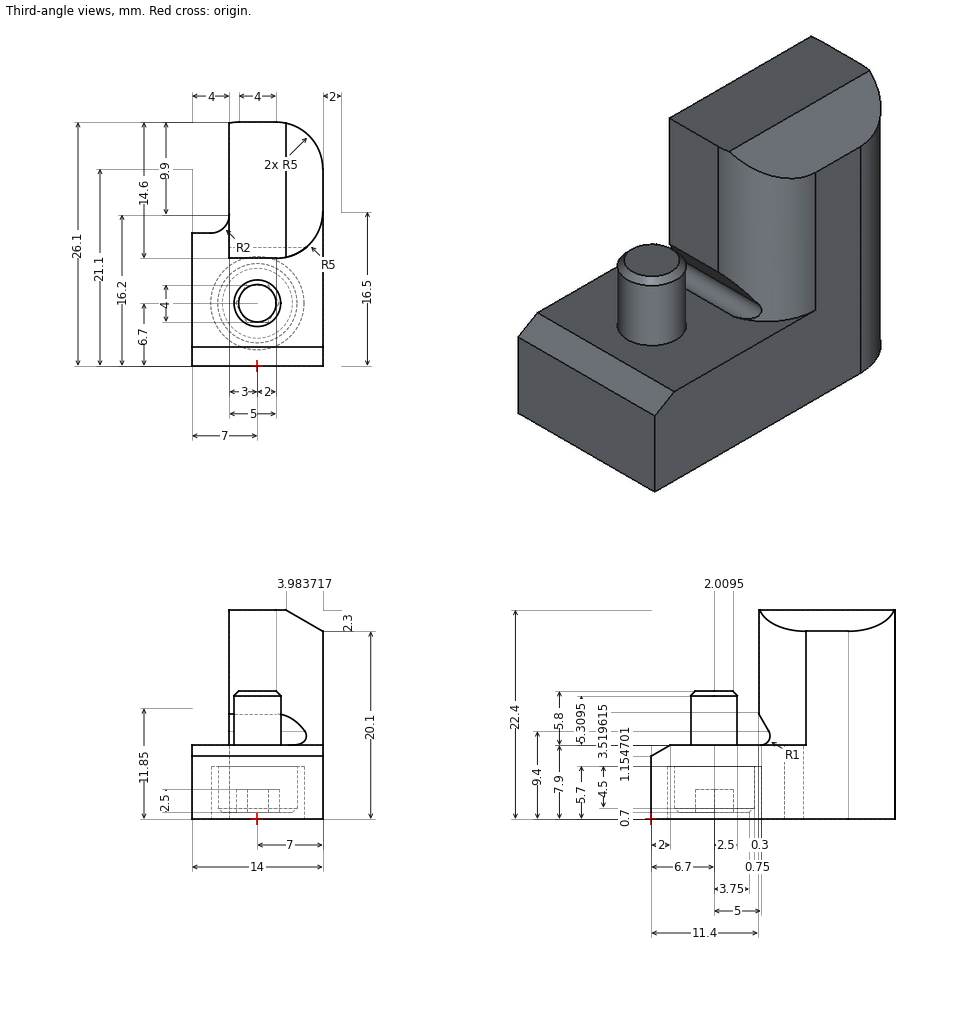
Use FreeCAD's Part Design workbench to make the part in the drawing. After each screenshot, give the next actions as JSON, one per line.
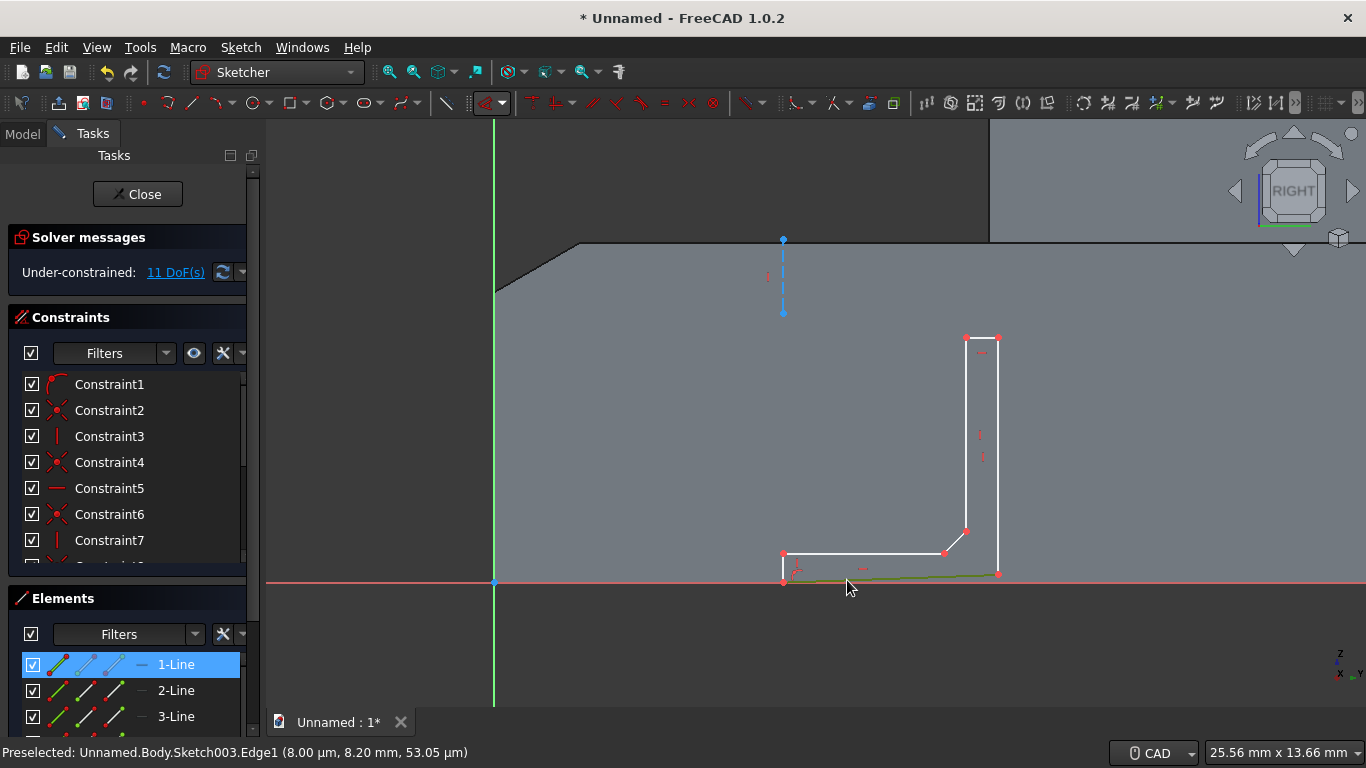
{"action": "key", "text": "h"}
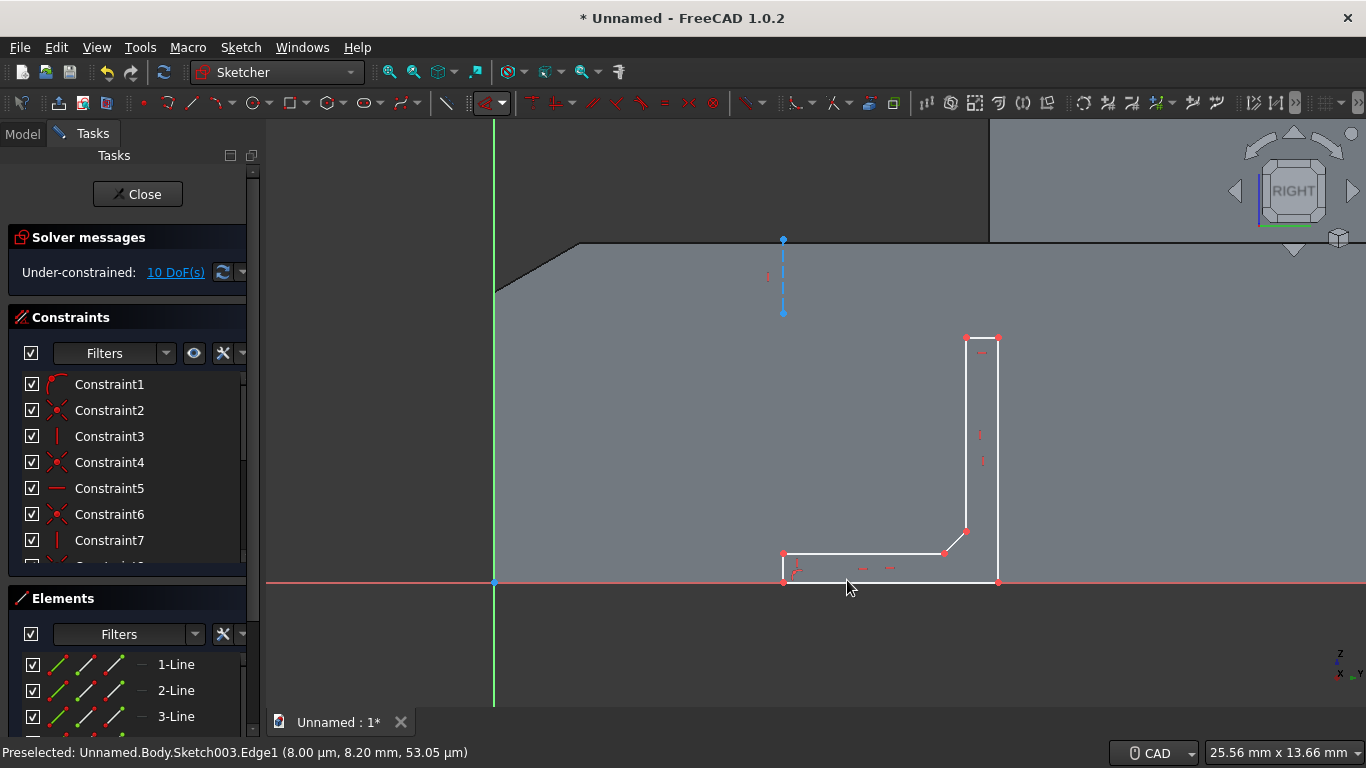
{"action": "left_click", "coordinate": [847, 583]}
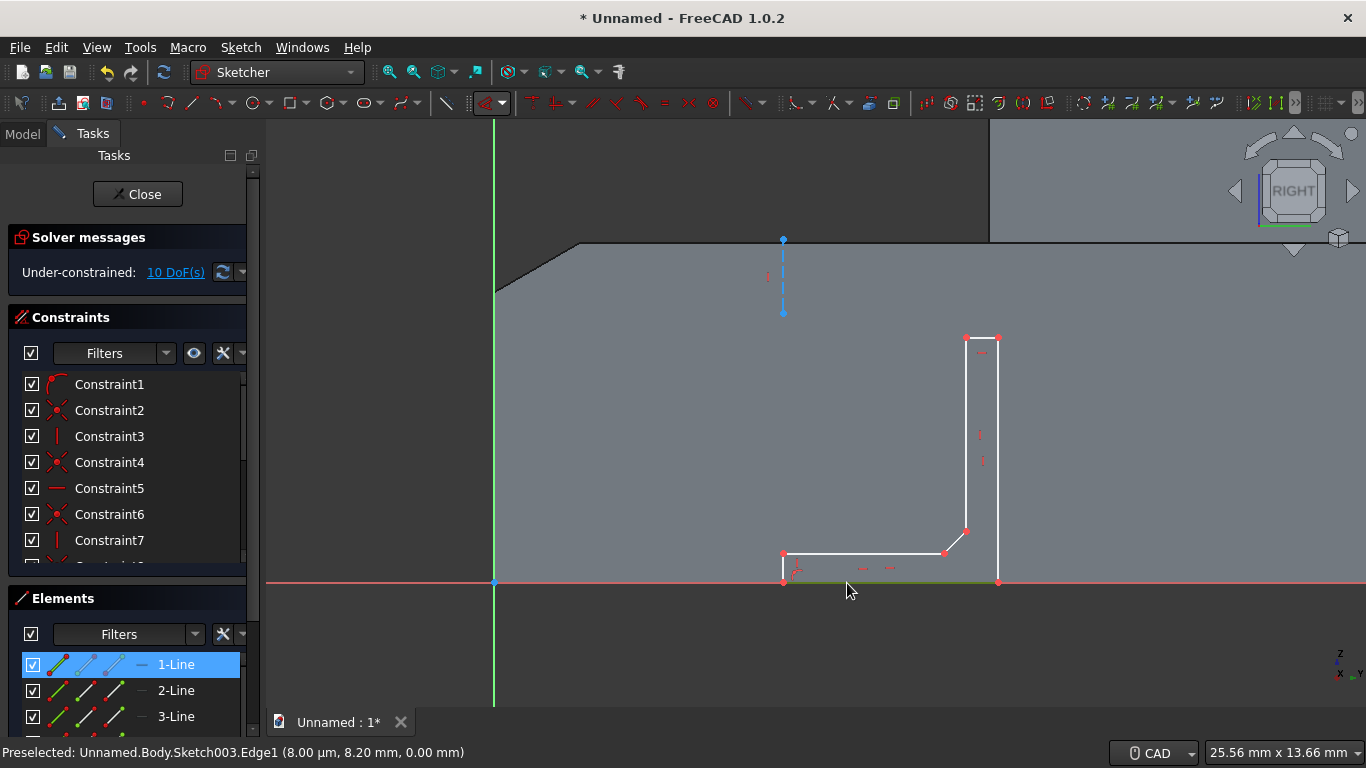
{"action": "key", "text": "l"}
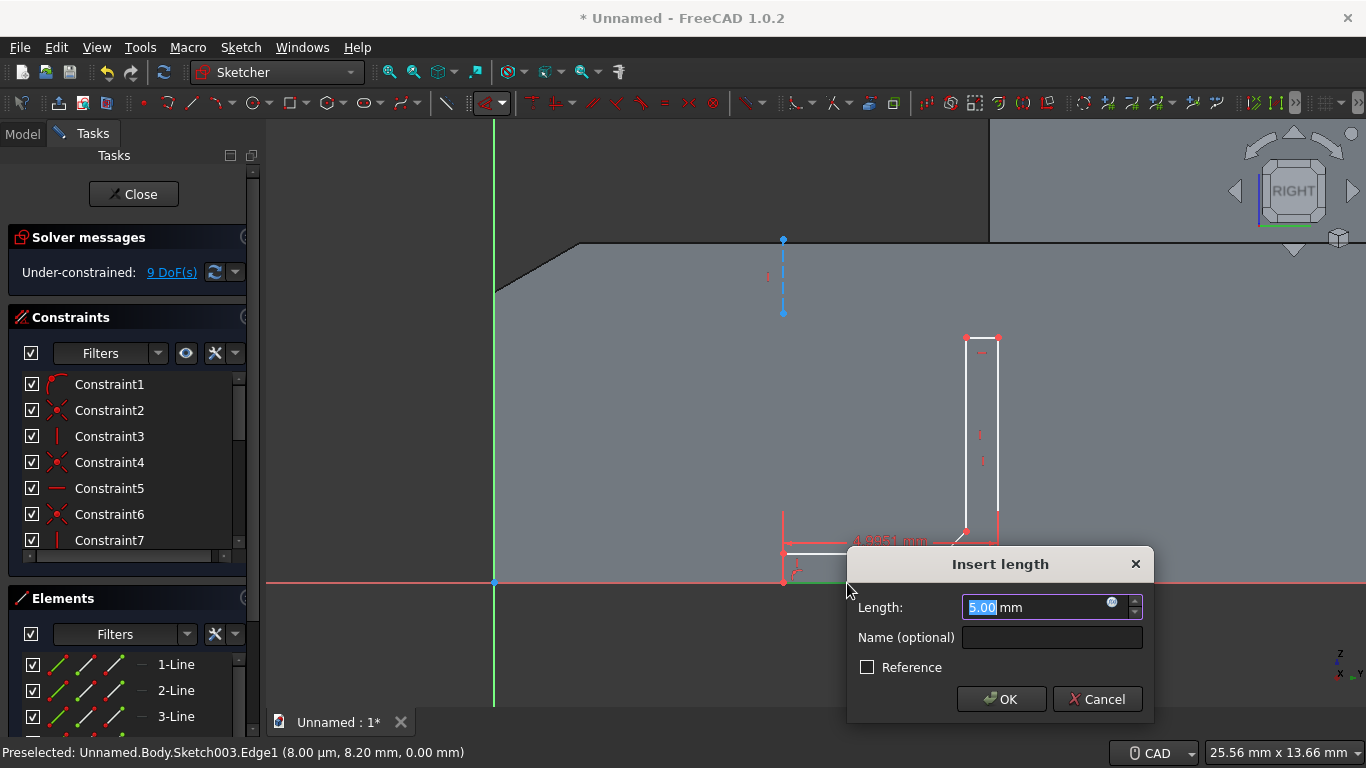
{"action": "type", "text": "5"}
{"action": "key", "text": "Return"}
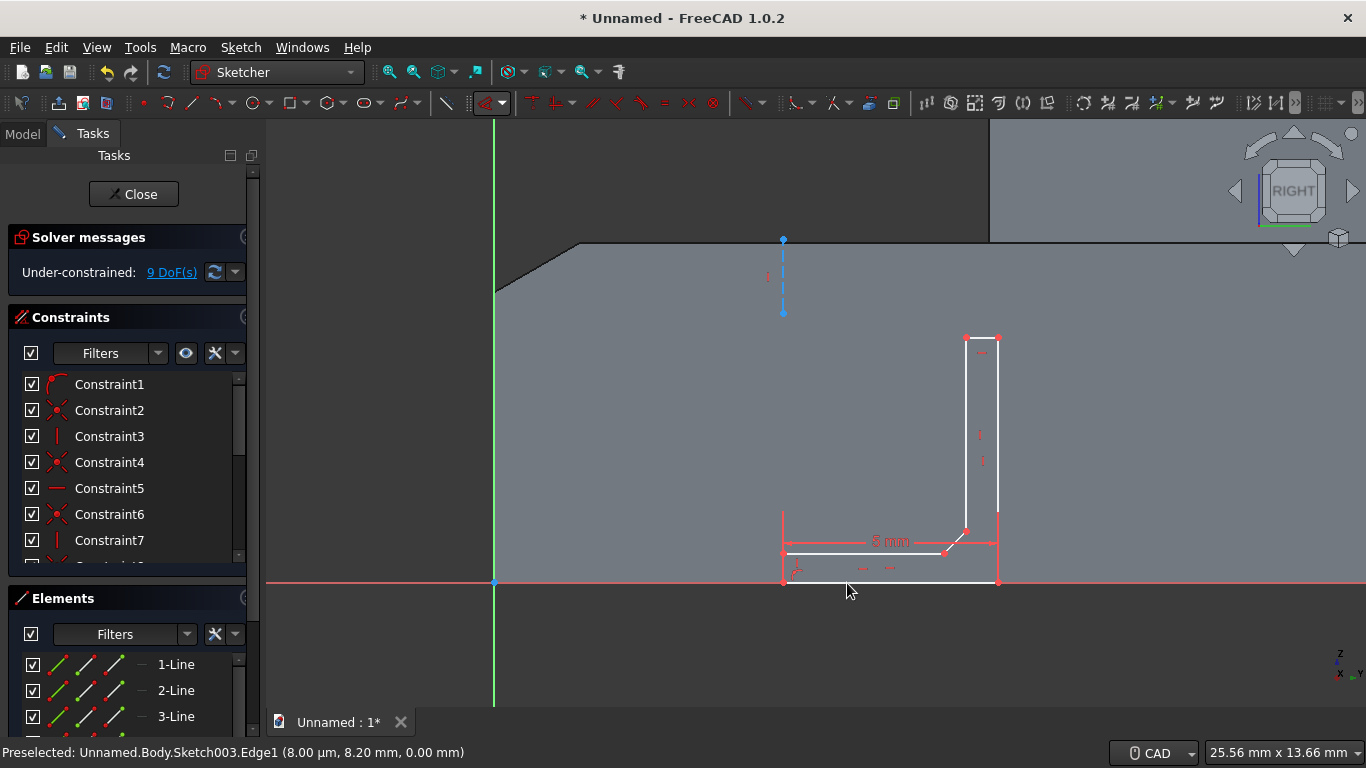
{"action": "left_click", "coordinate": [998, 509]}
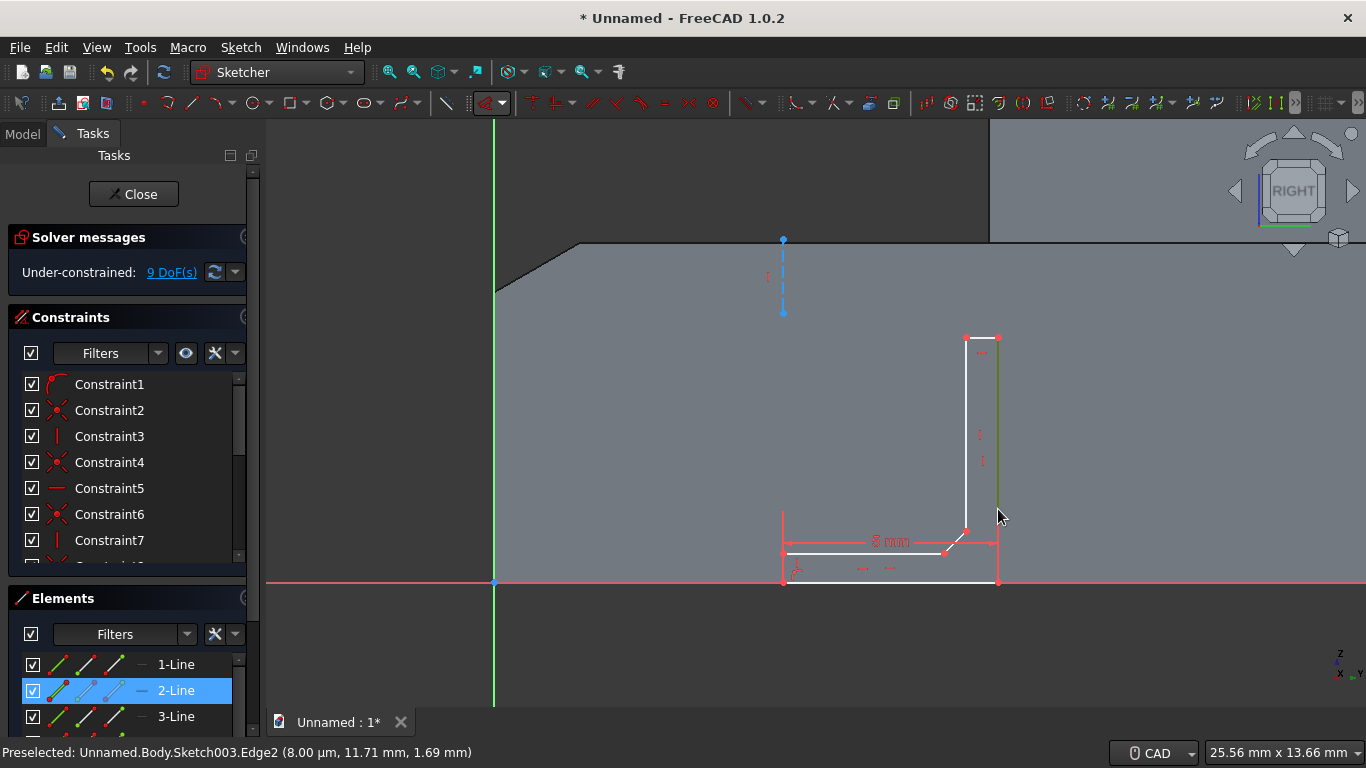
{"action": "left_click", "coordinate": [504, 104]}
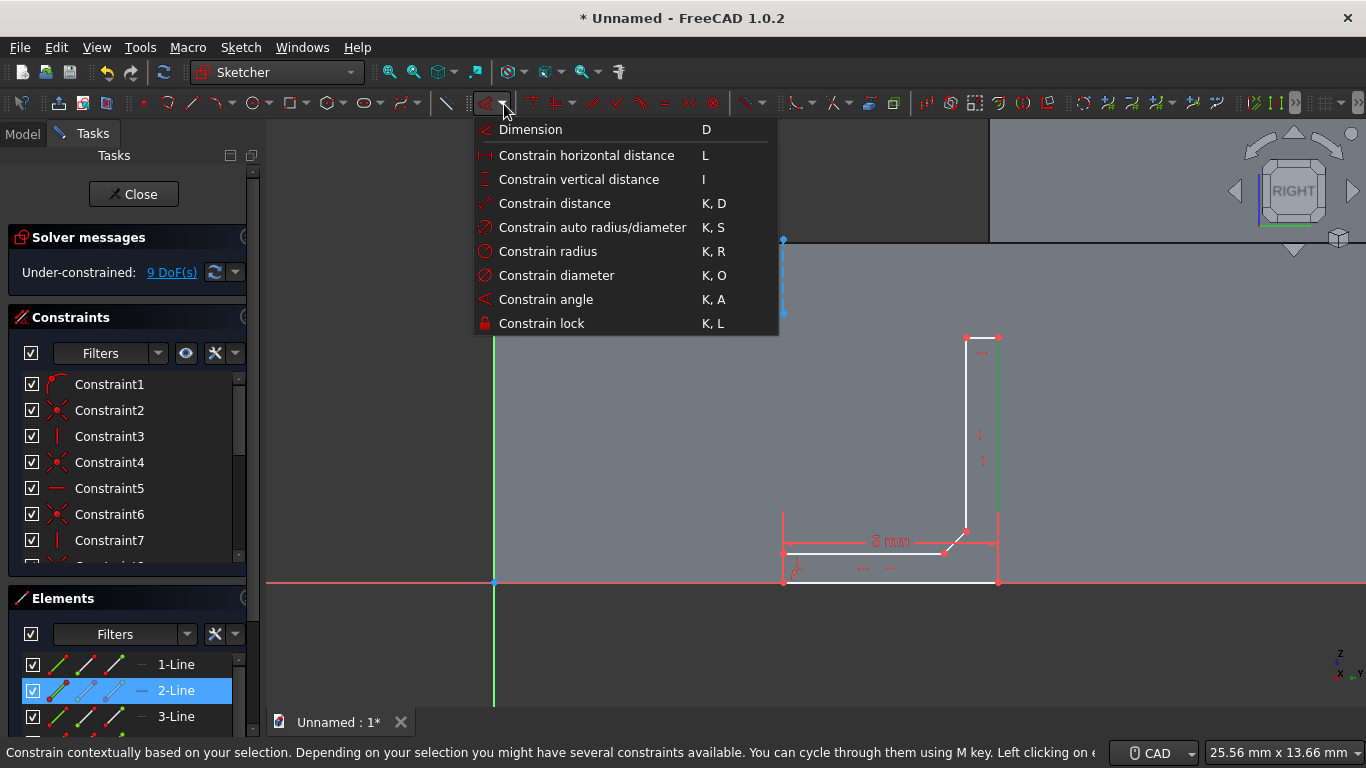
{"action": "left_click", "coordinate": [626, 179]}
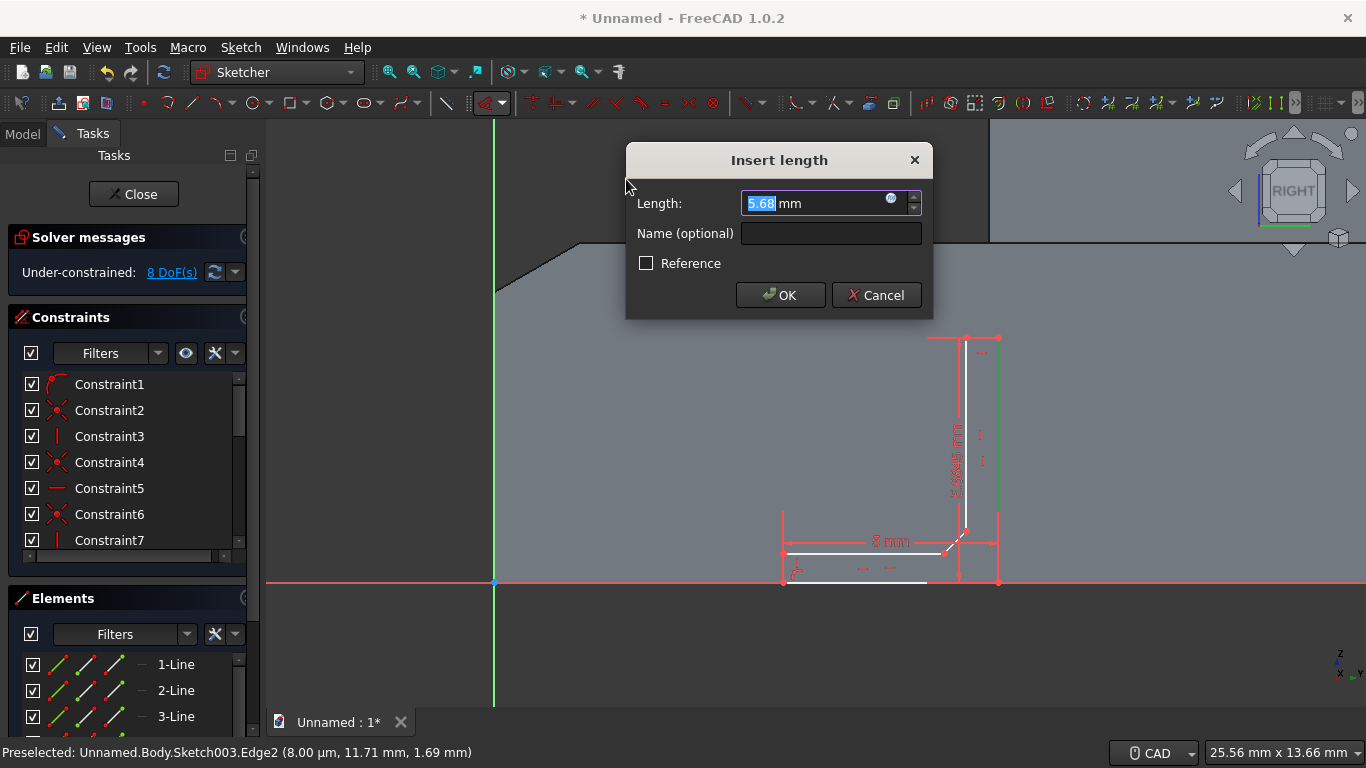
{"action": "type", "text": "5.7"}
{"action": "key", "text": "Return"}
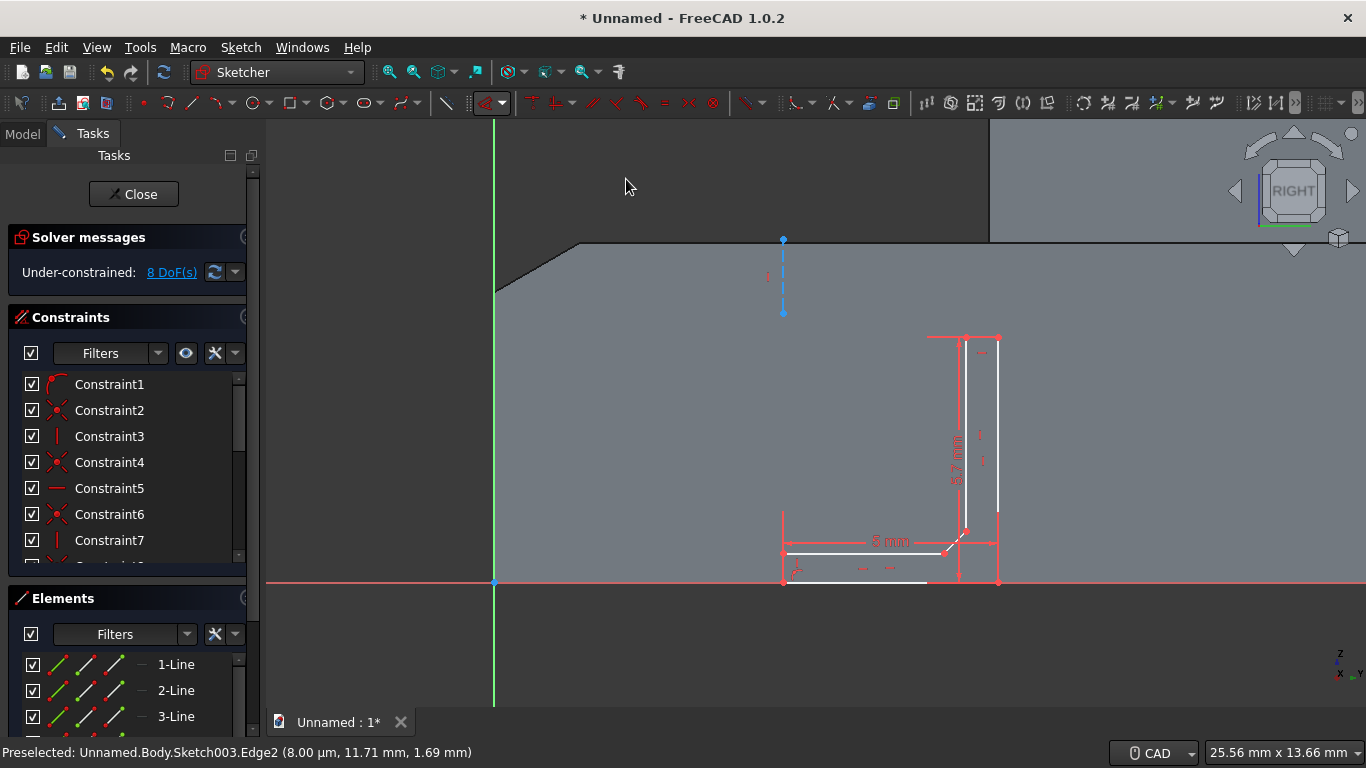
{"action": "left_click", "coordinate": [966, 396]}